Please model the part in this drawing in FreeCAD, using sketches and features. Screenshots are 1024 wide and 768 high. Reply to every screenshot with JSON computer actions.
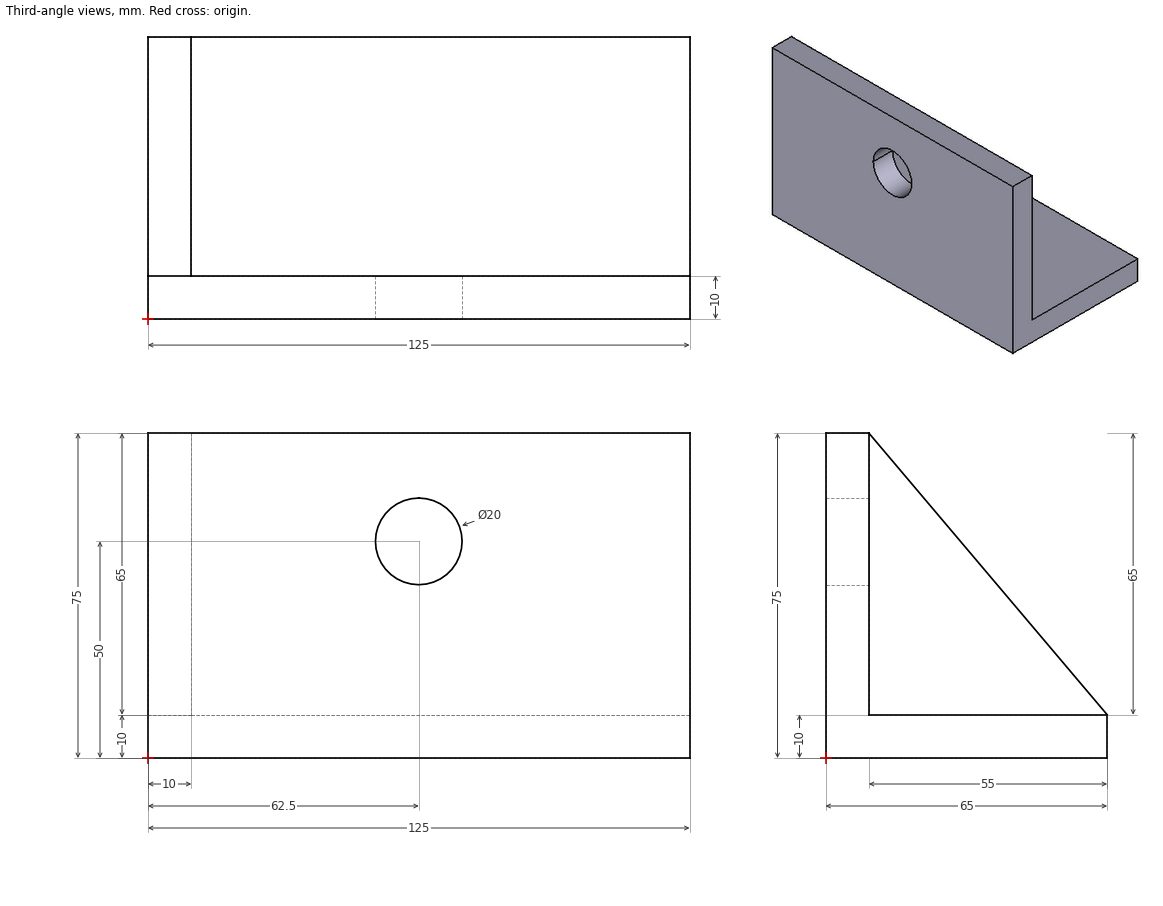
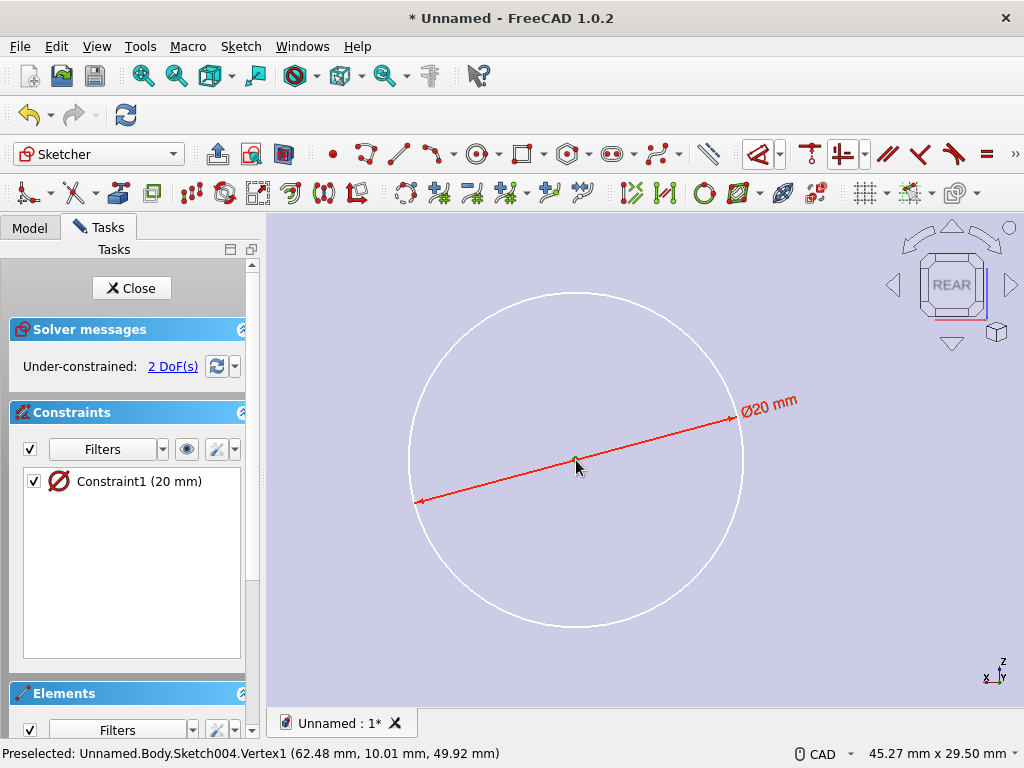
{"action": "key", "text": "i"}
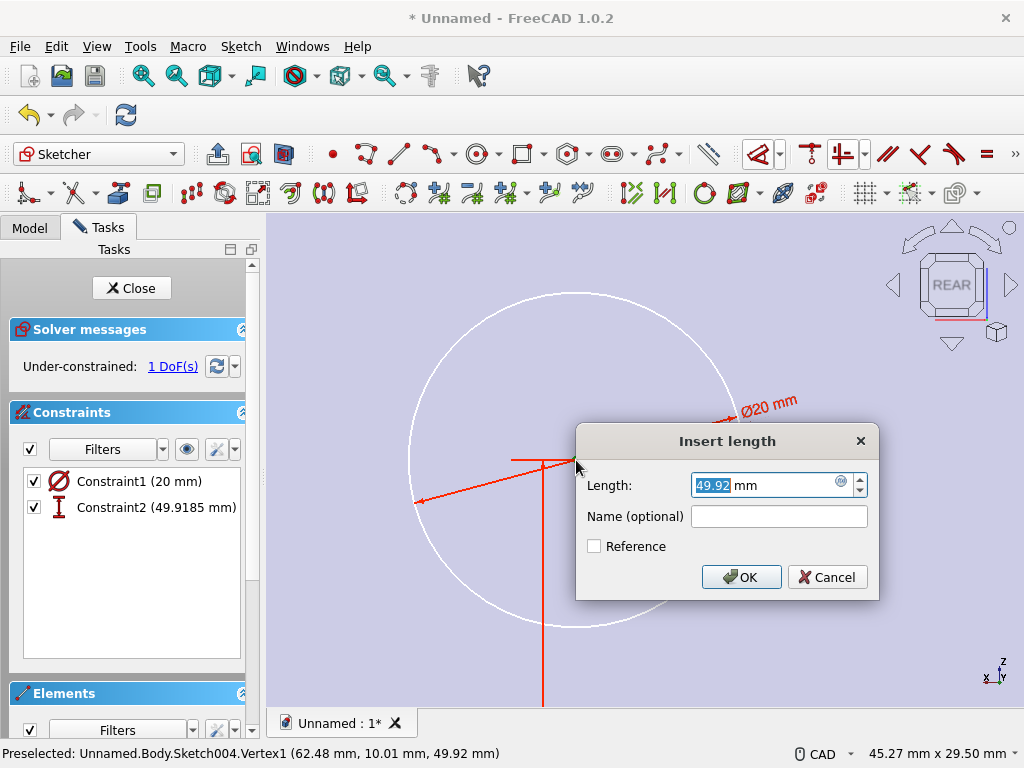
{"action": "type", "text": "50"}
{"action": "key", "text": "Return"}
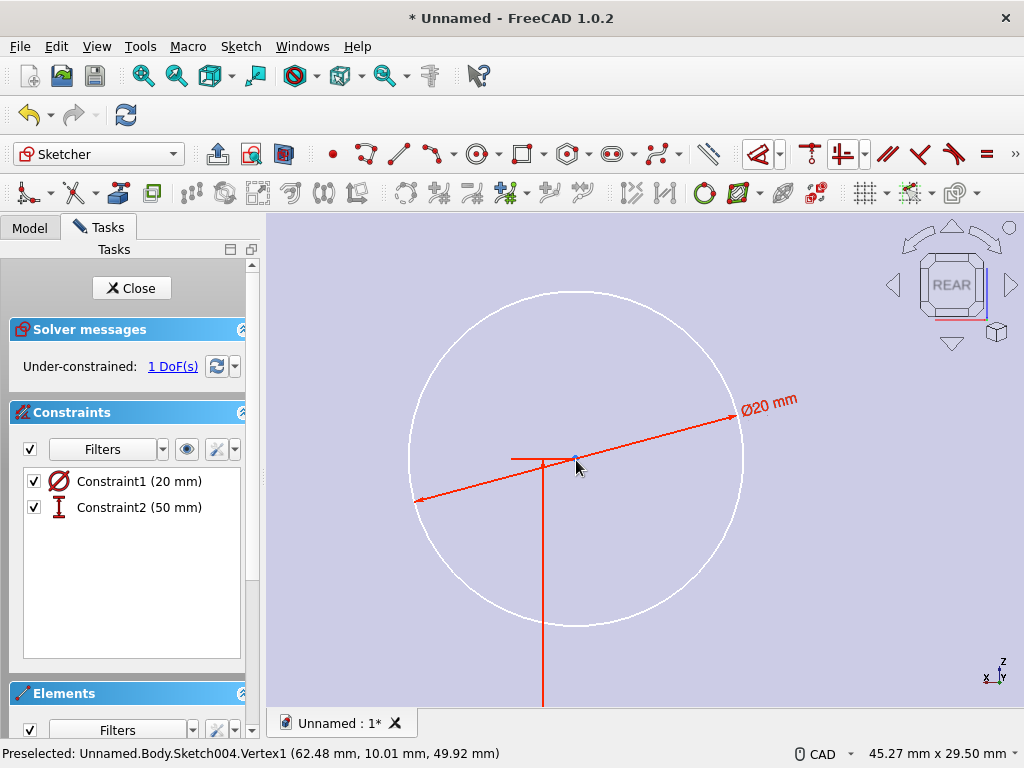
{"action": "left_click", "coordinate": [576, 459]}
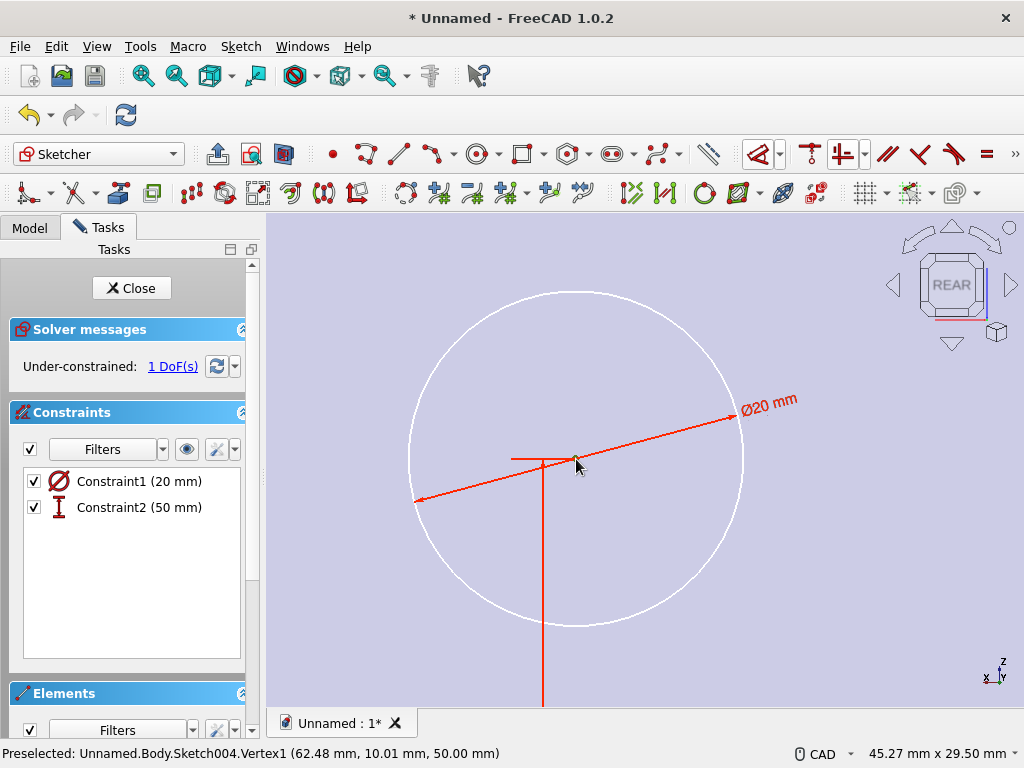
{"action": "key", "text": "l"}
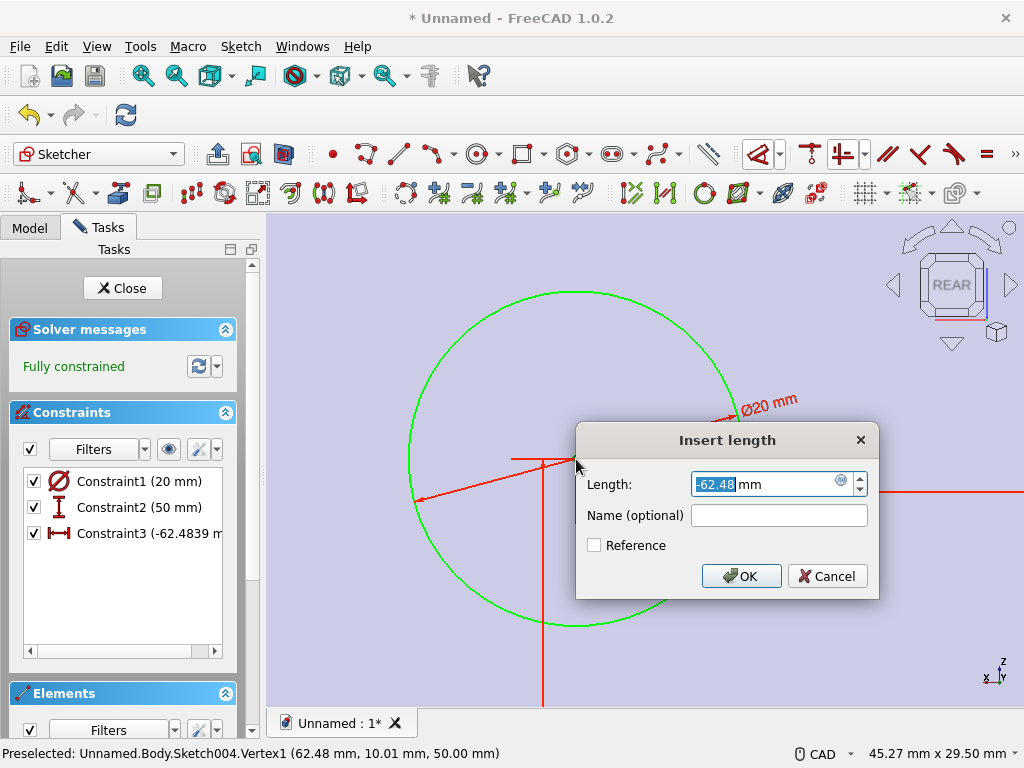
{"action": "type", "text": "-62.5"}
{"action": "key", "text": "Return"}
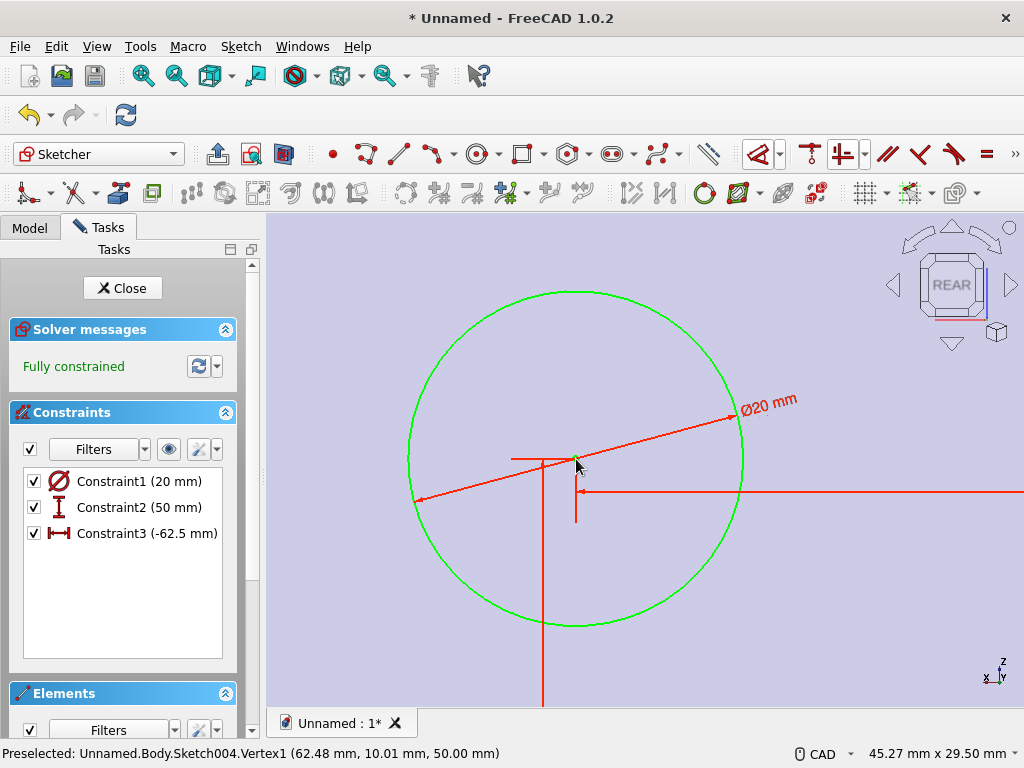
{"action": "left_click", "coordinate": [123, 288]}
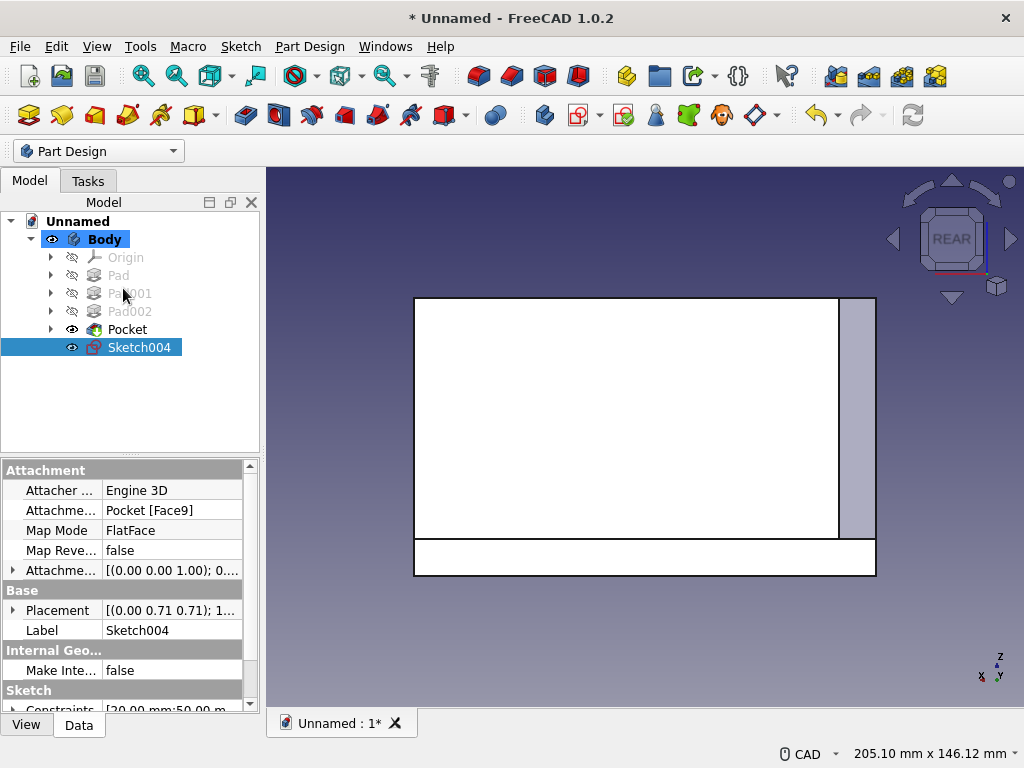
{"action": "left_click", "coordinate": [246, 116]}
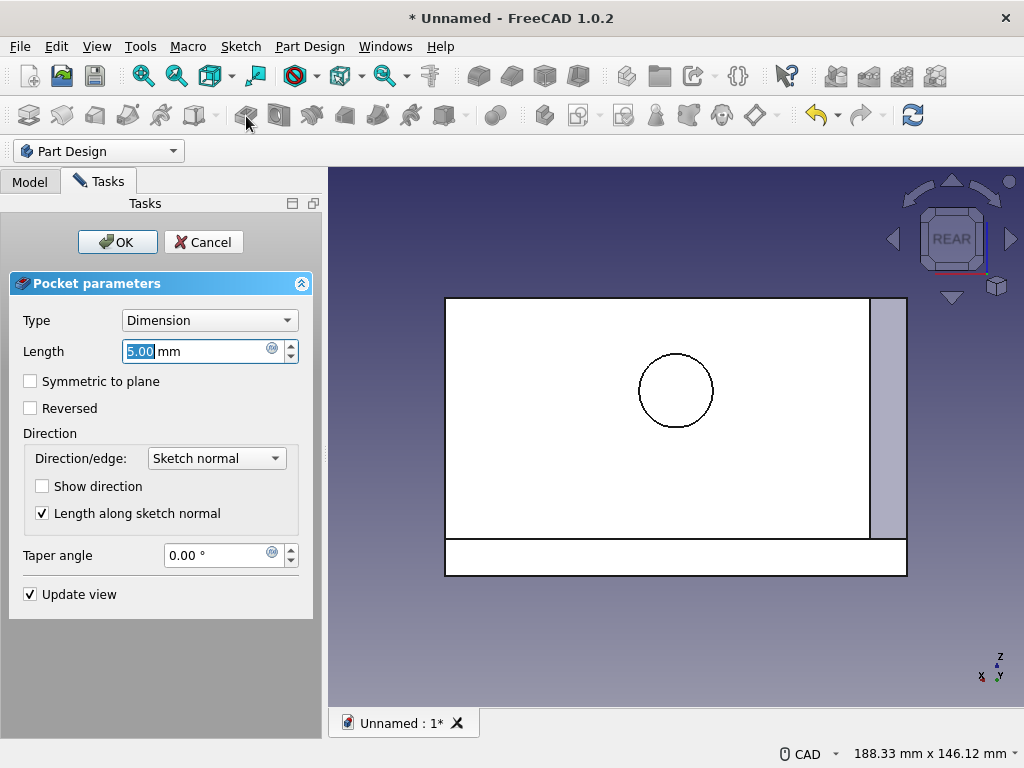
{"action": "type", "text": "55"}
{"action": "key", "text": "Tab"}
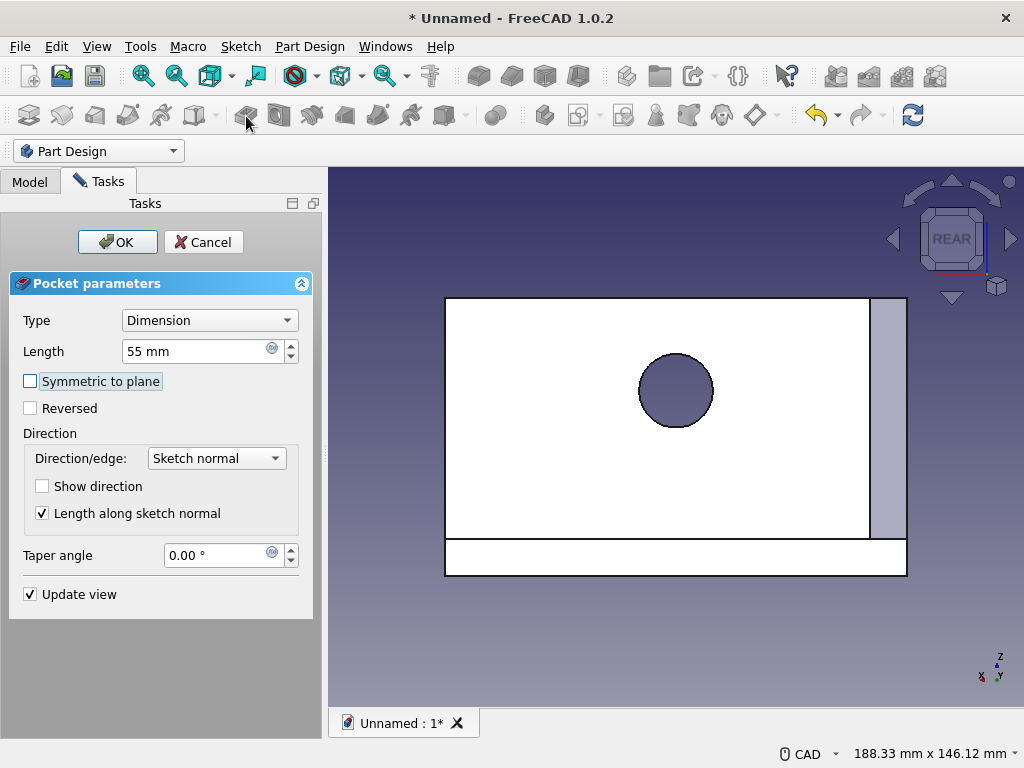
{"action": "left_click", "coordinate": [118, 242]}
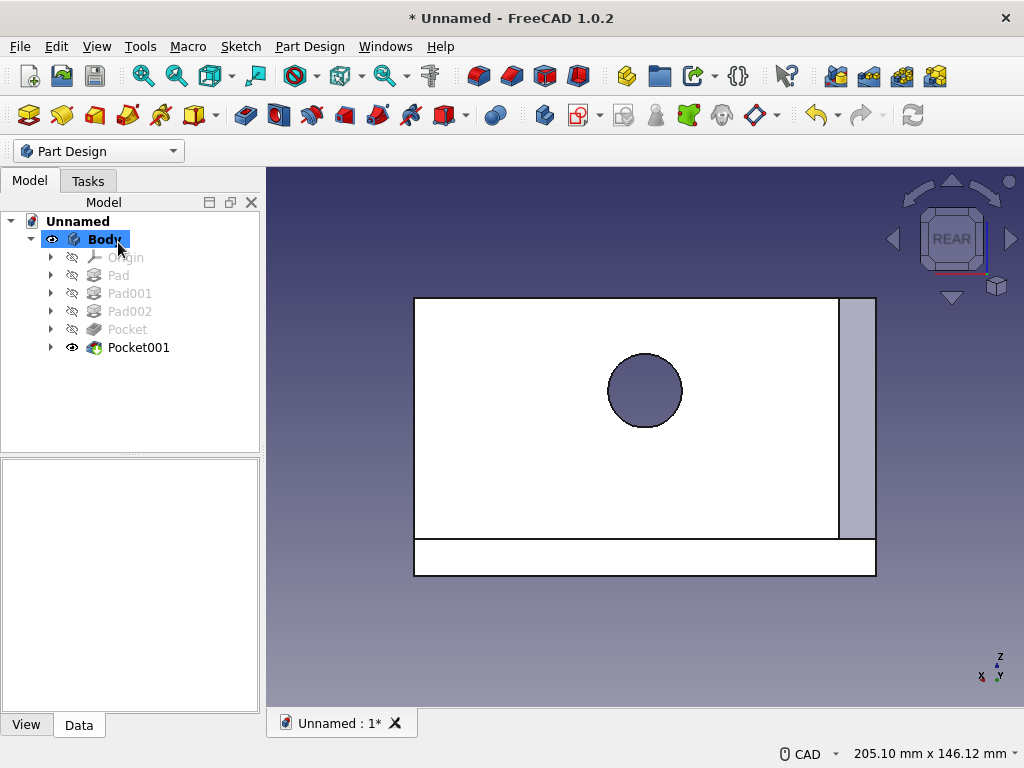
{"action": "key", "text": "0"}